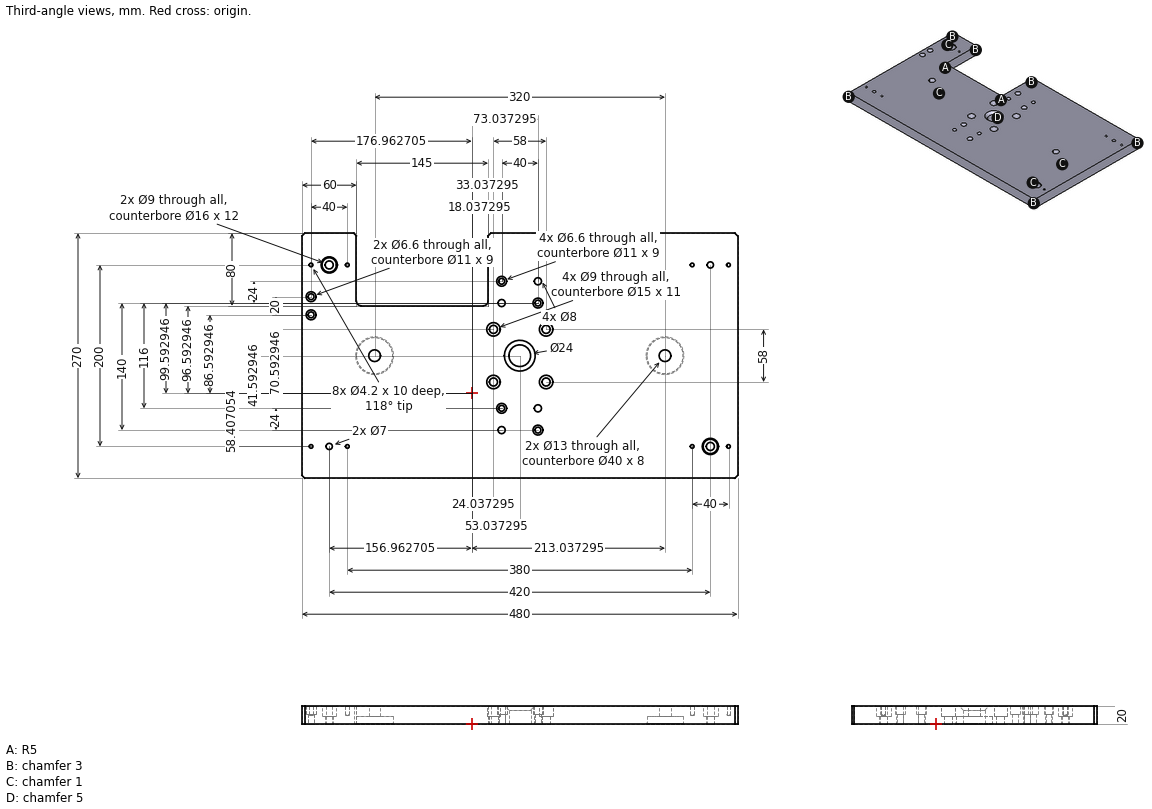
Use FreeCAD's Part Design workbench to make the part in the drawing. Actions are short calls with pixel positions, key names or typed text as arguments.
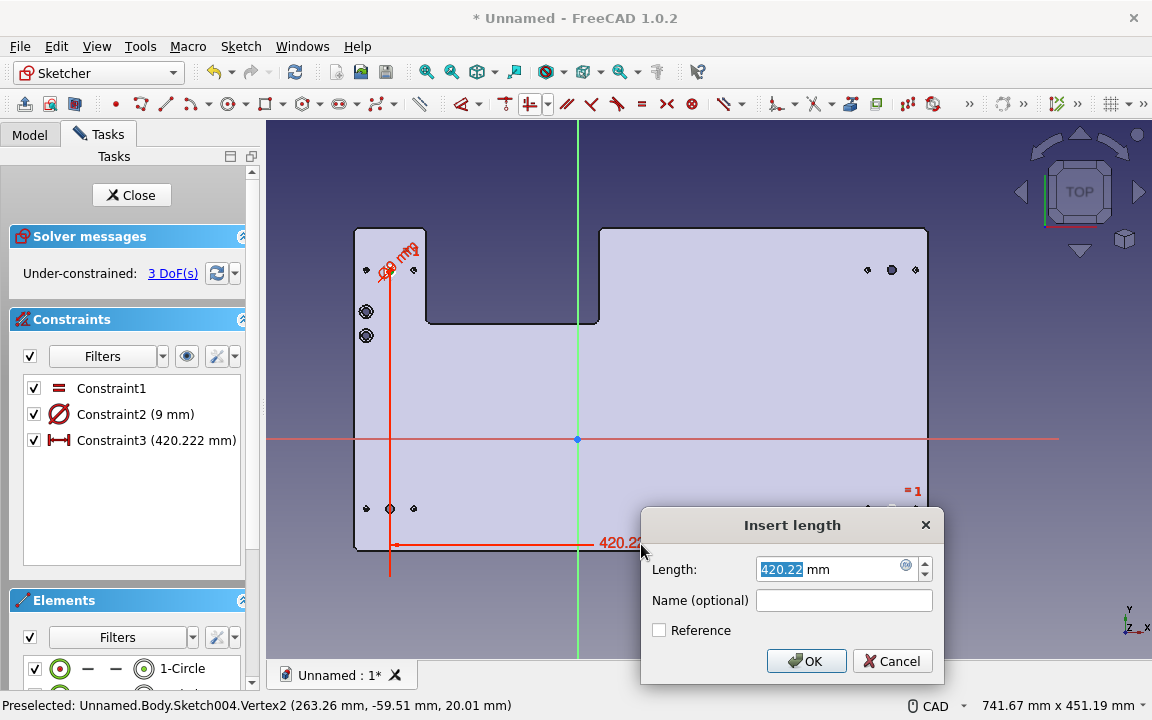
text(420)
key(Return)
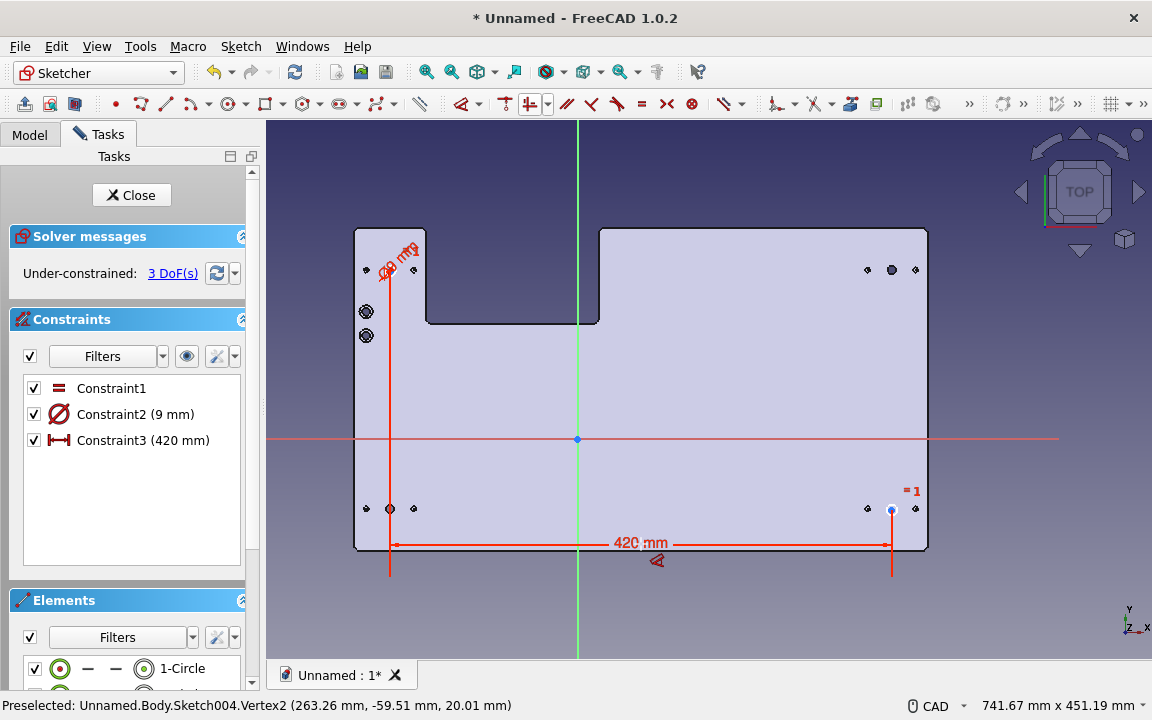
click(390, 271)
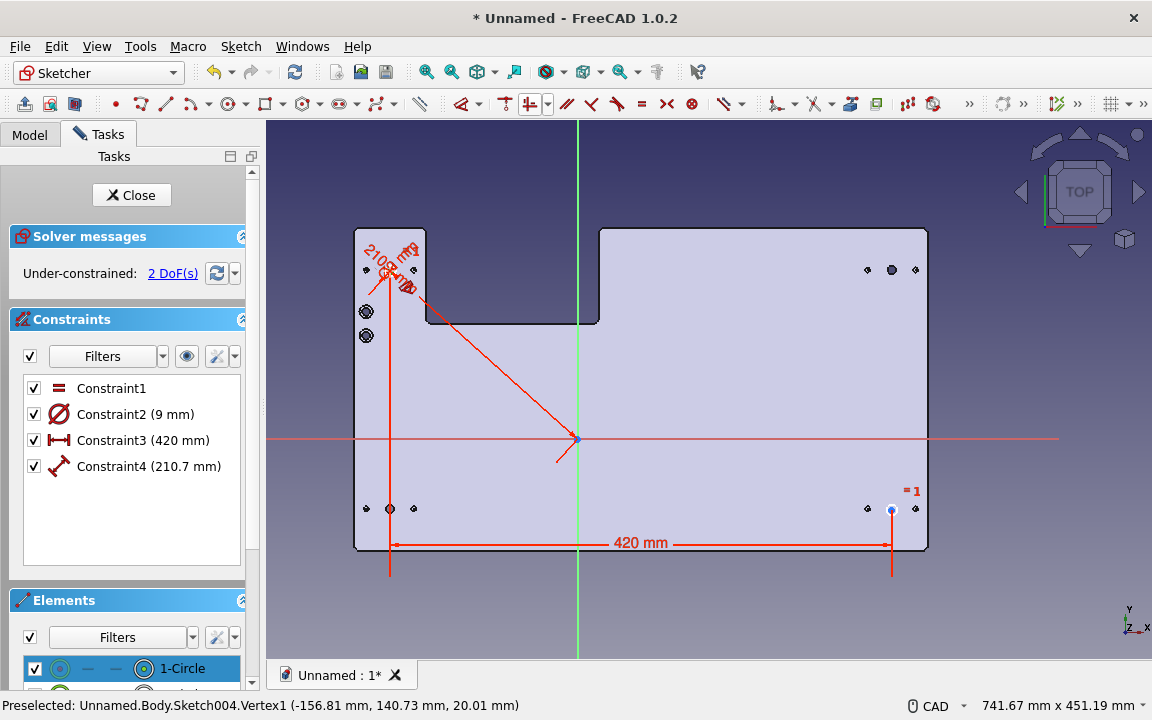
click(892, 510)
click(926, 391)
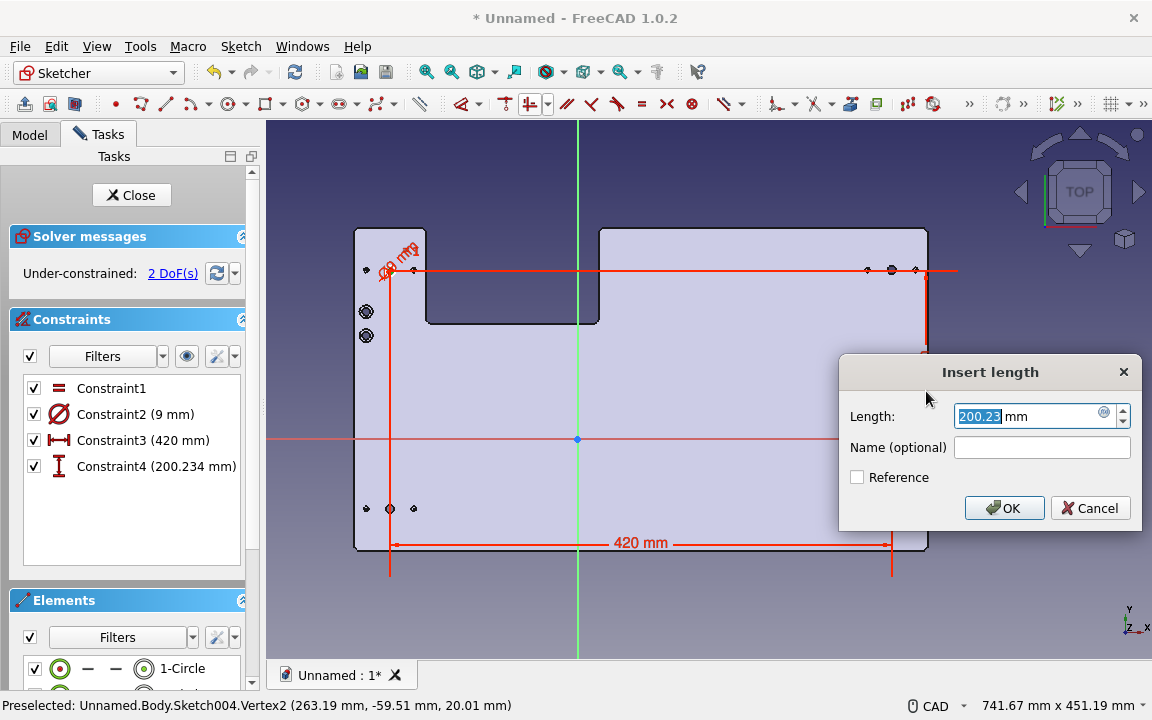
text(200)
key(Return)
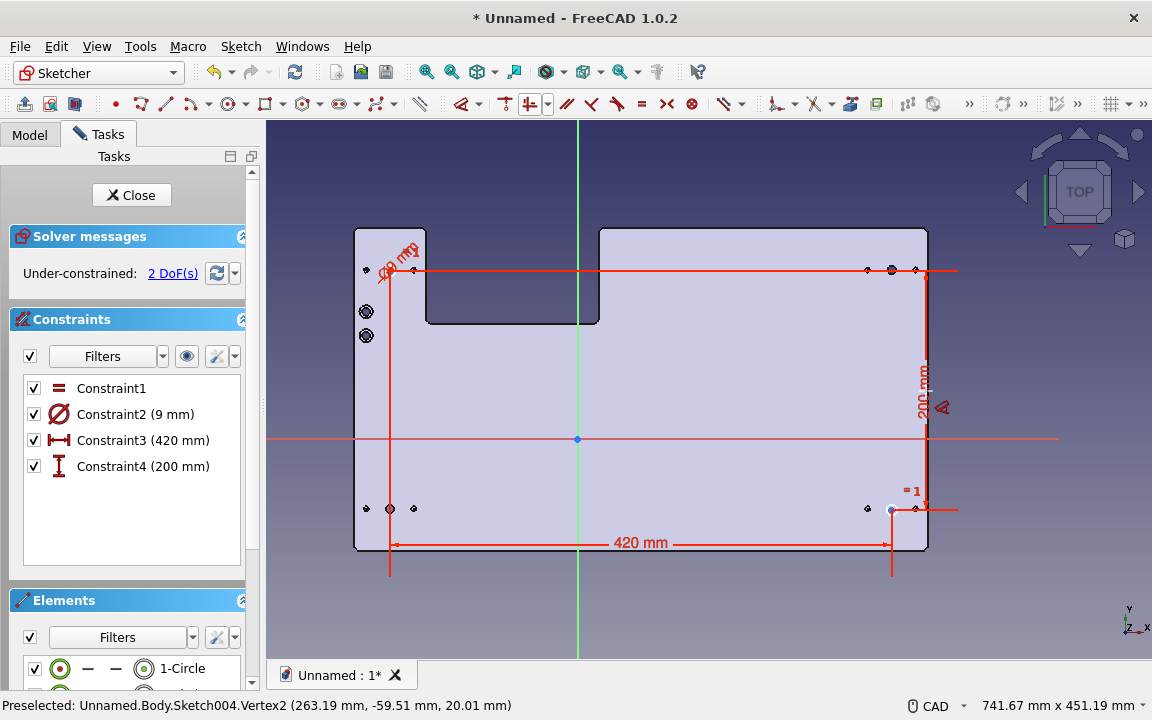
click(892, 510)
click(926, 475)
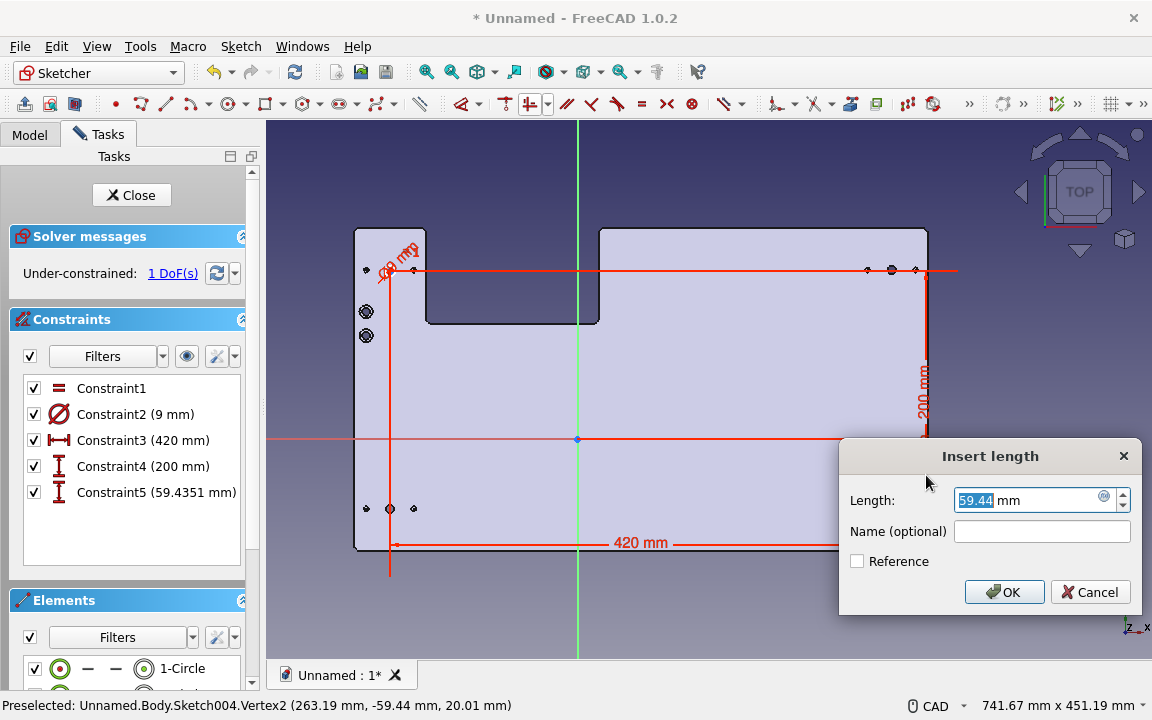
text(58.407054)
key(Return)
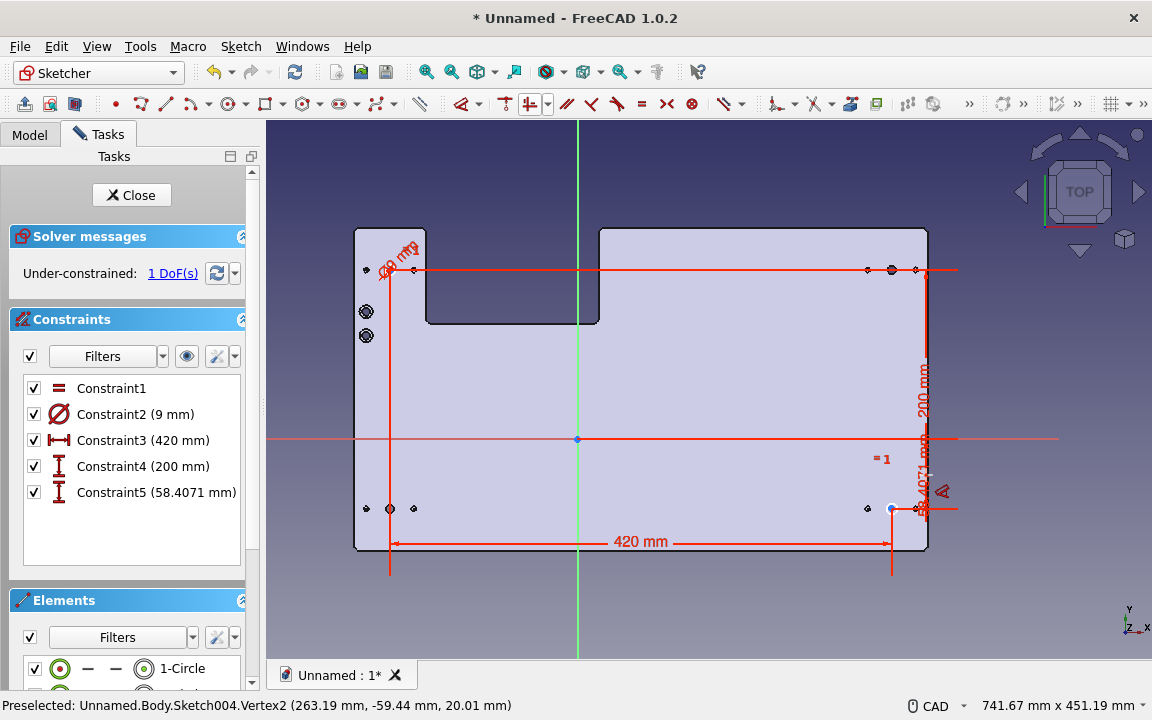
click(390, 270)
click(484, 236)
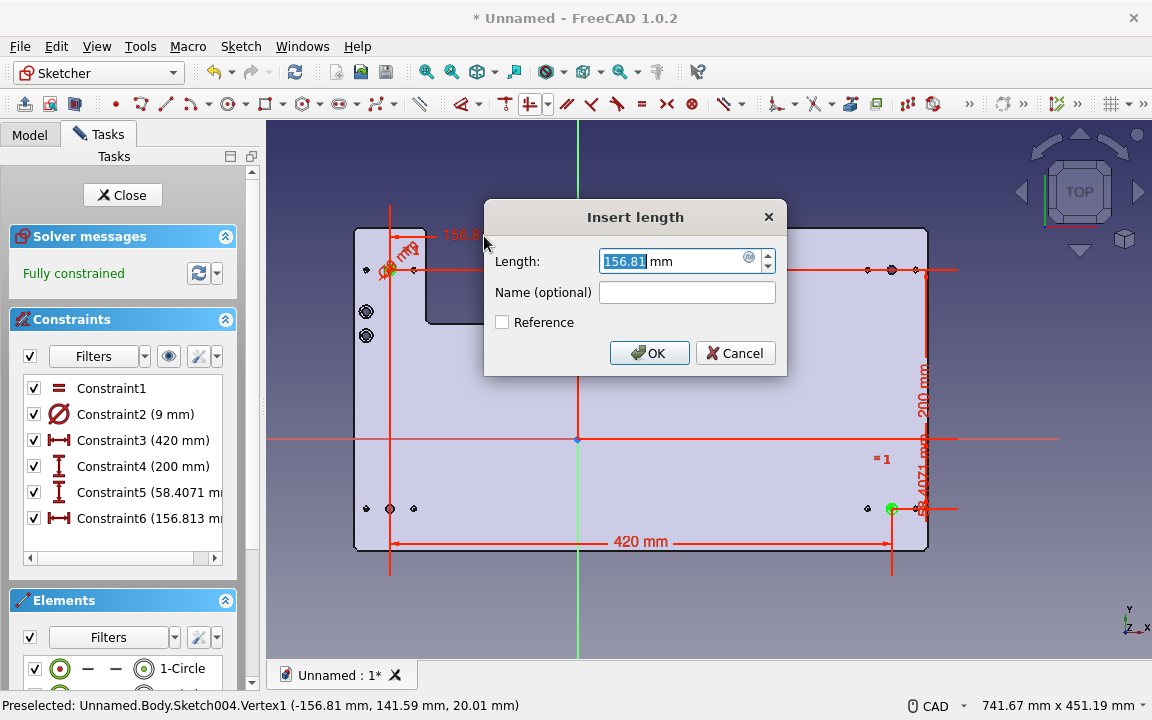
text(156.962705)
key(Return)
key(Escape)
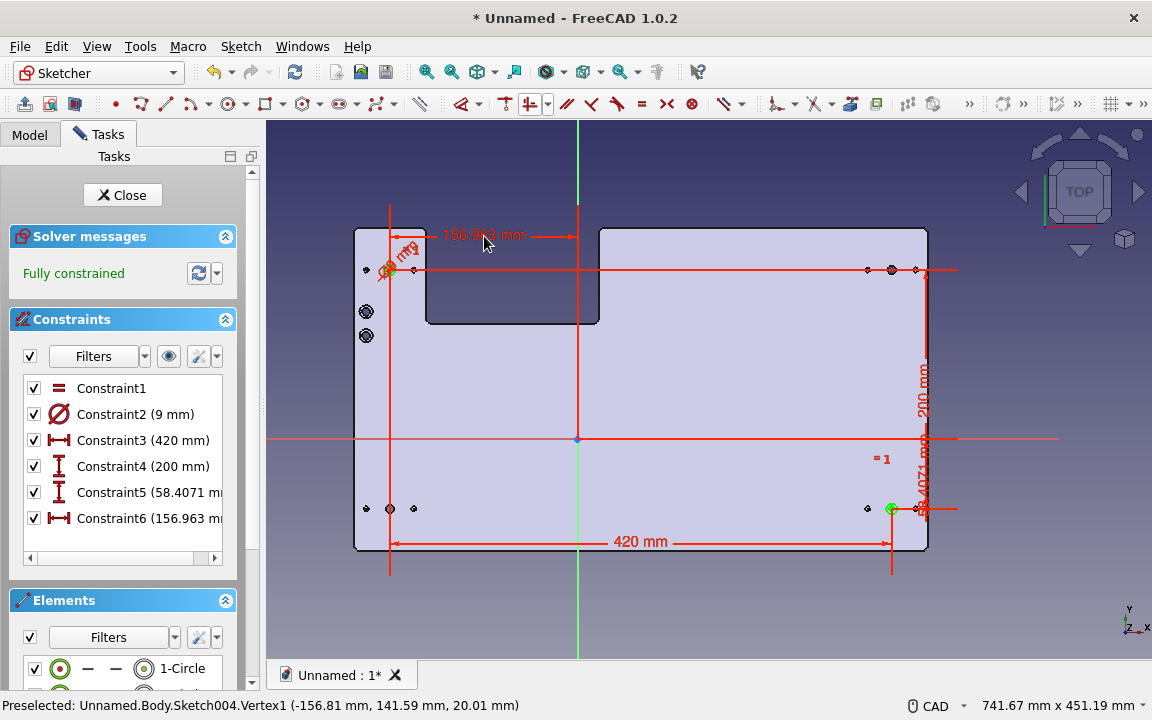
click(123, 195)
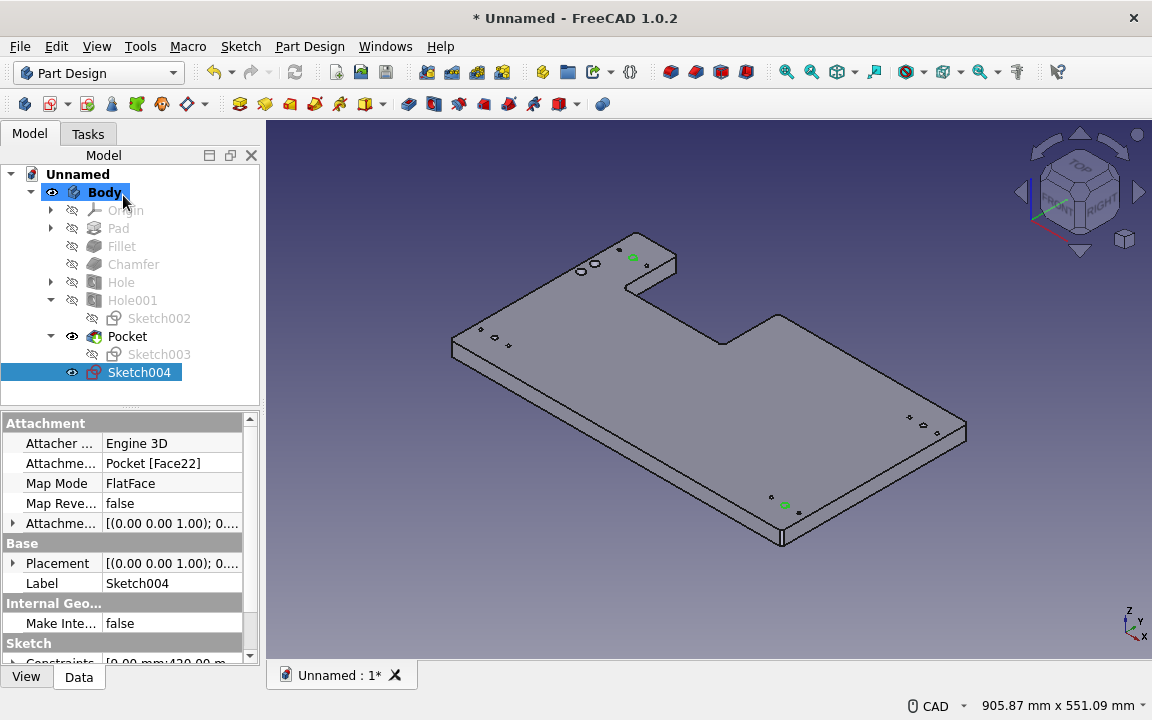
click(434, 104)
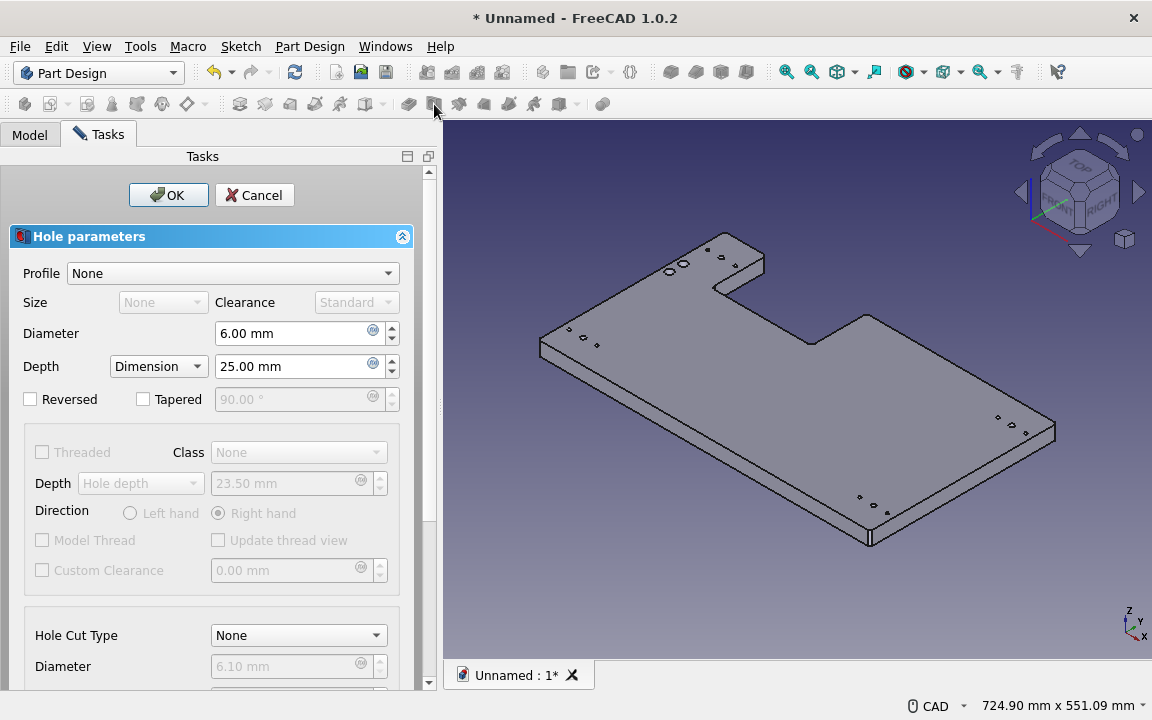
triple_click(300, 334)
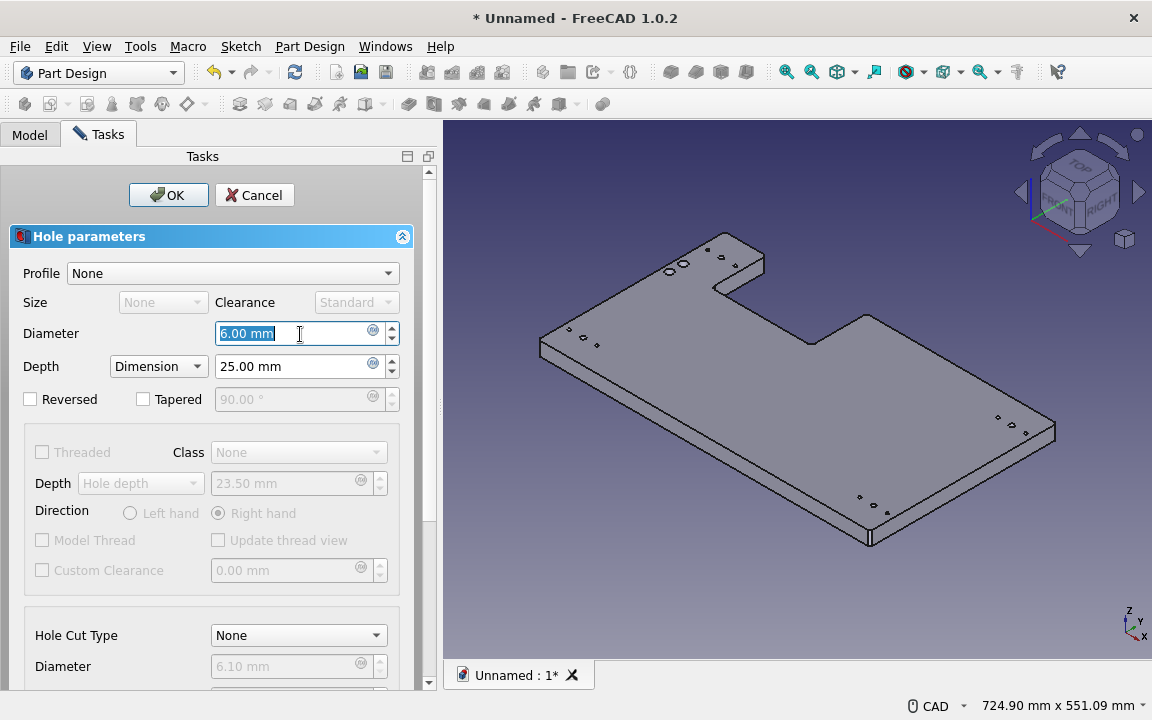
text(9)
key(Tab)